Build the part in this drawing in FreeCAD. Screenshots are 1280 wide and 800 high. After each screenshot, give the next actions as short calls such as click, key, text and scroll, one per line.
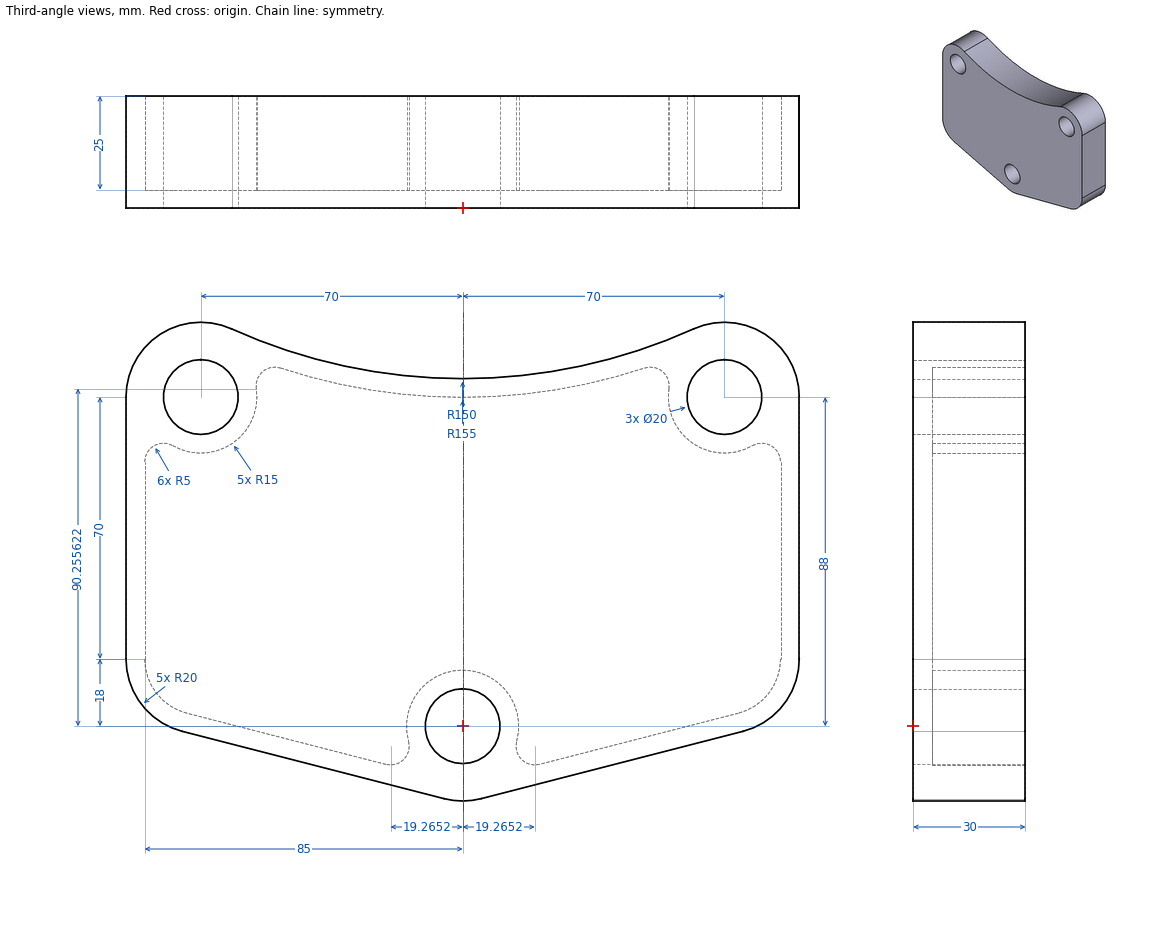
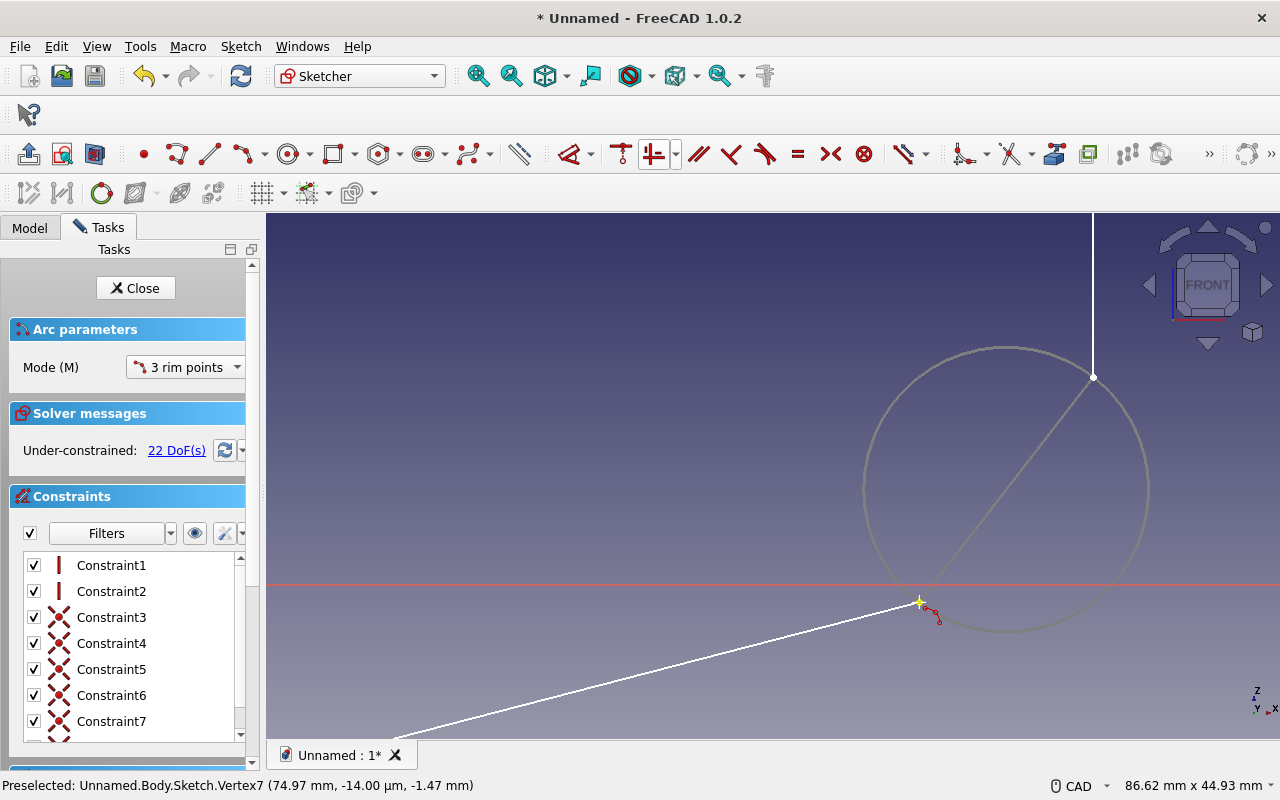
scroll(922, 605, down, 7)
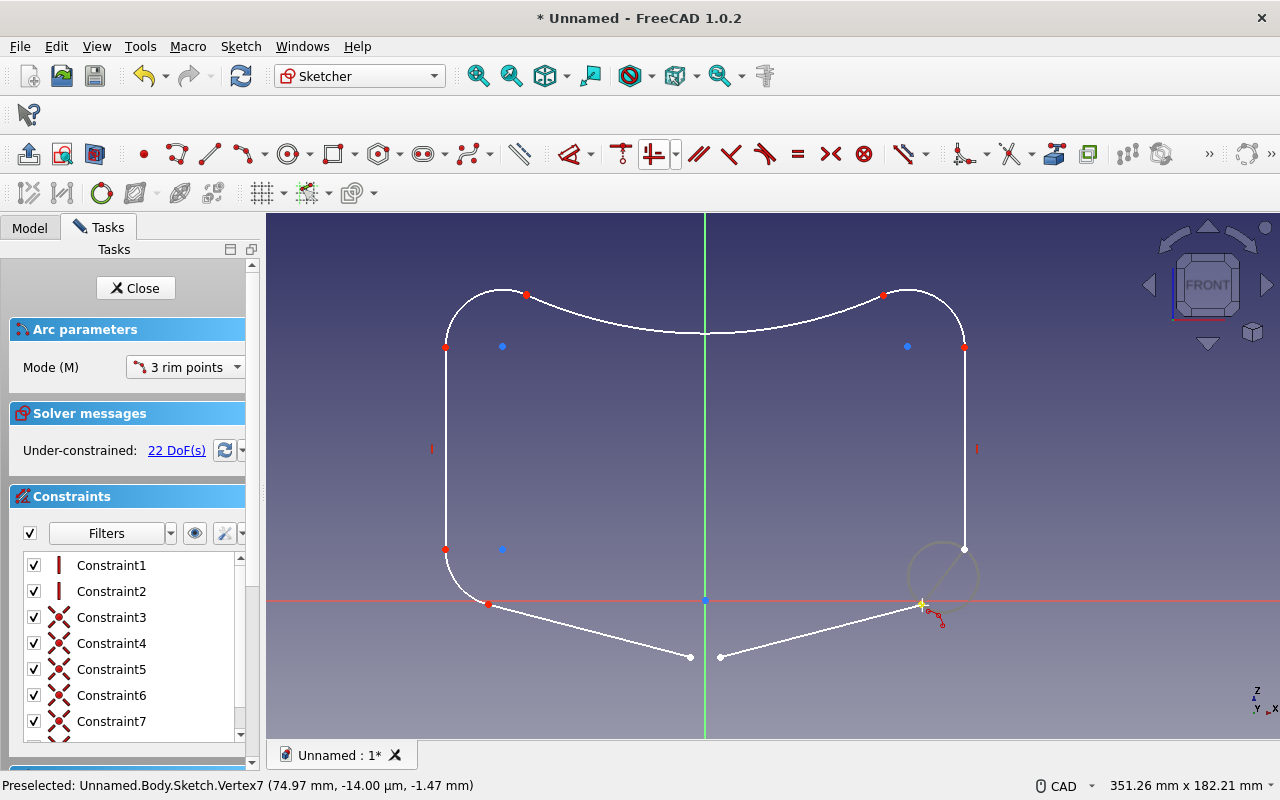
scroll(953, 584, up, 2)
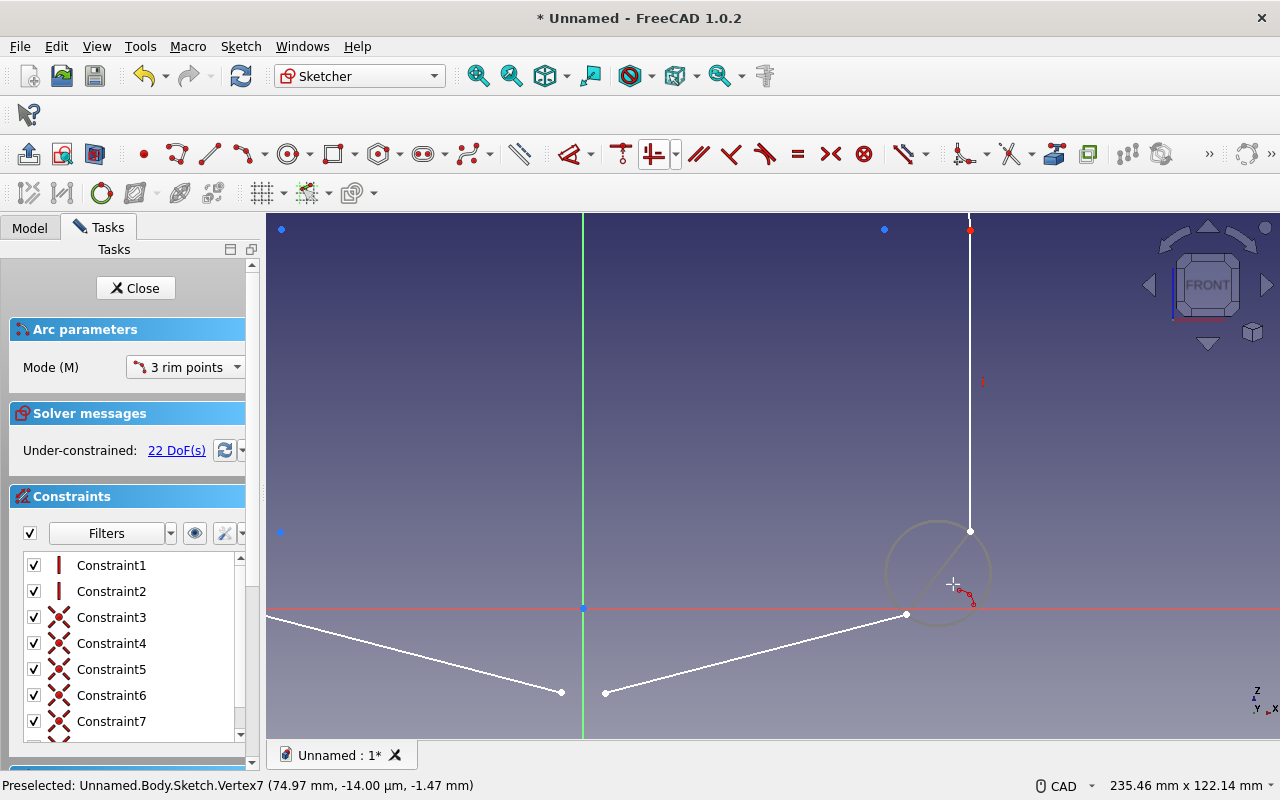
click(953, 584)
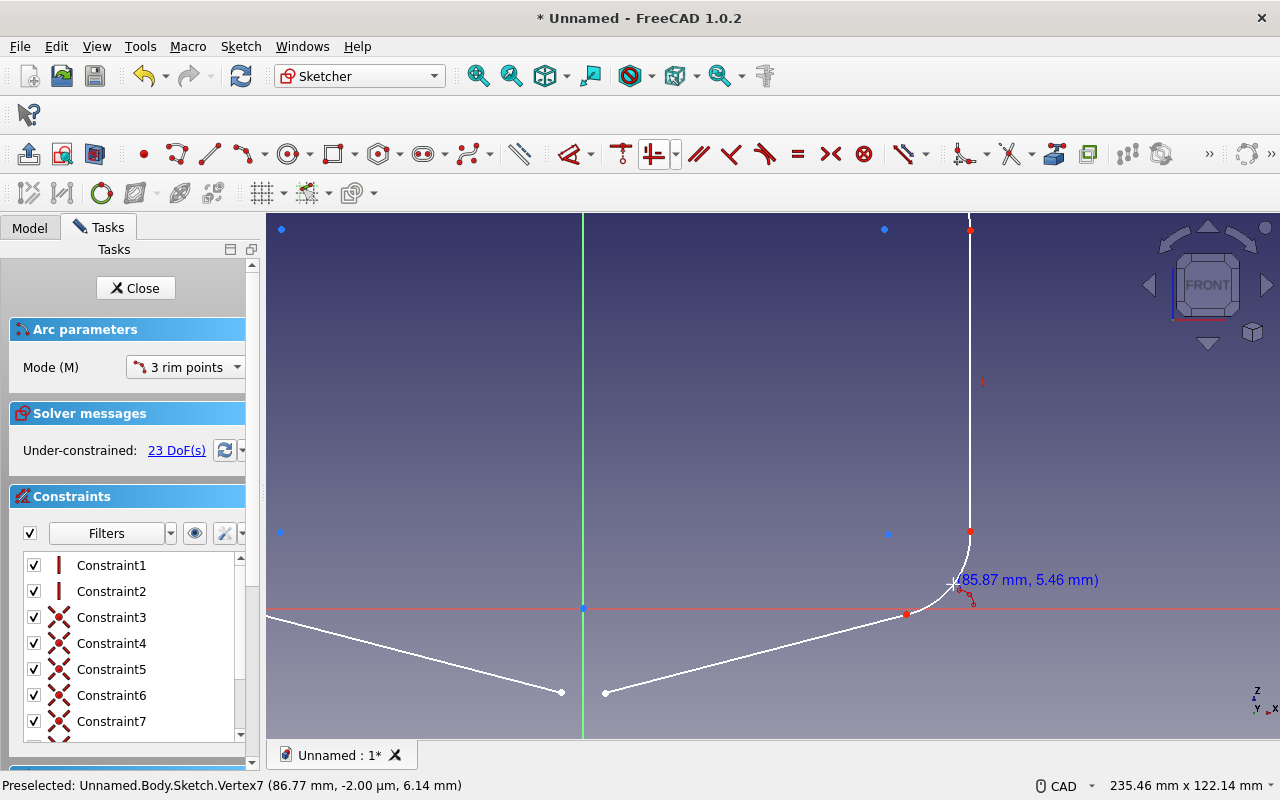
click(605, 693)
click(561, 693)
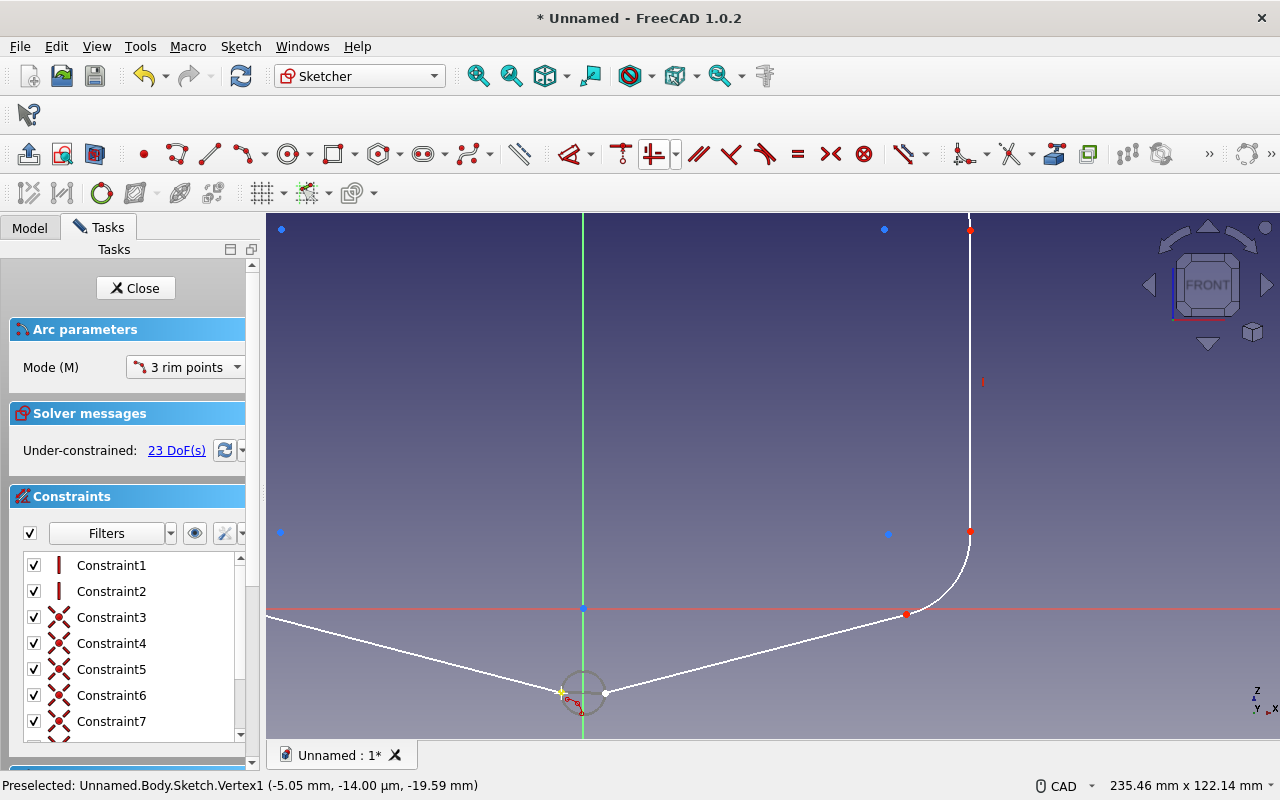
scroll(579, 695, up, 10)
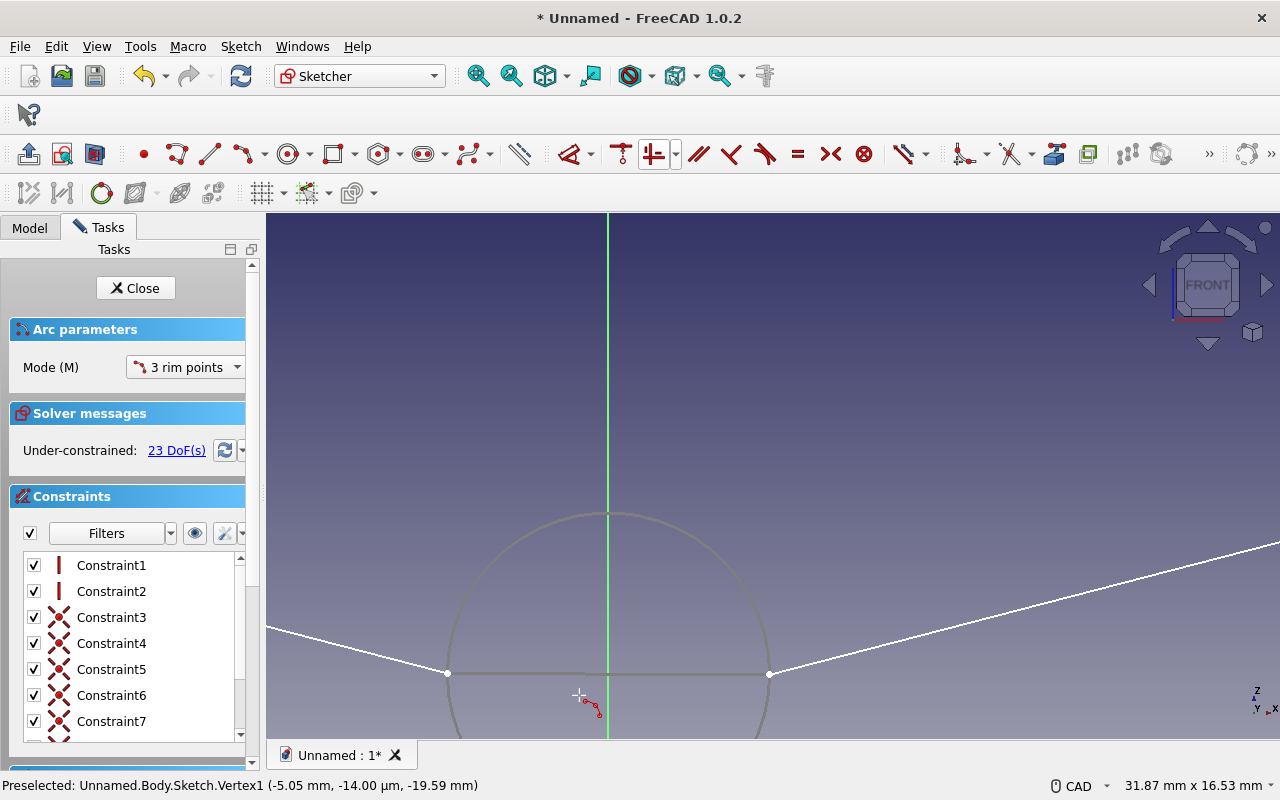
click(576, 686)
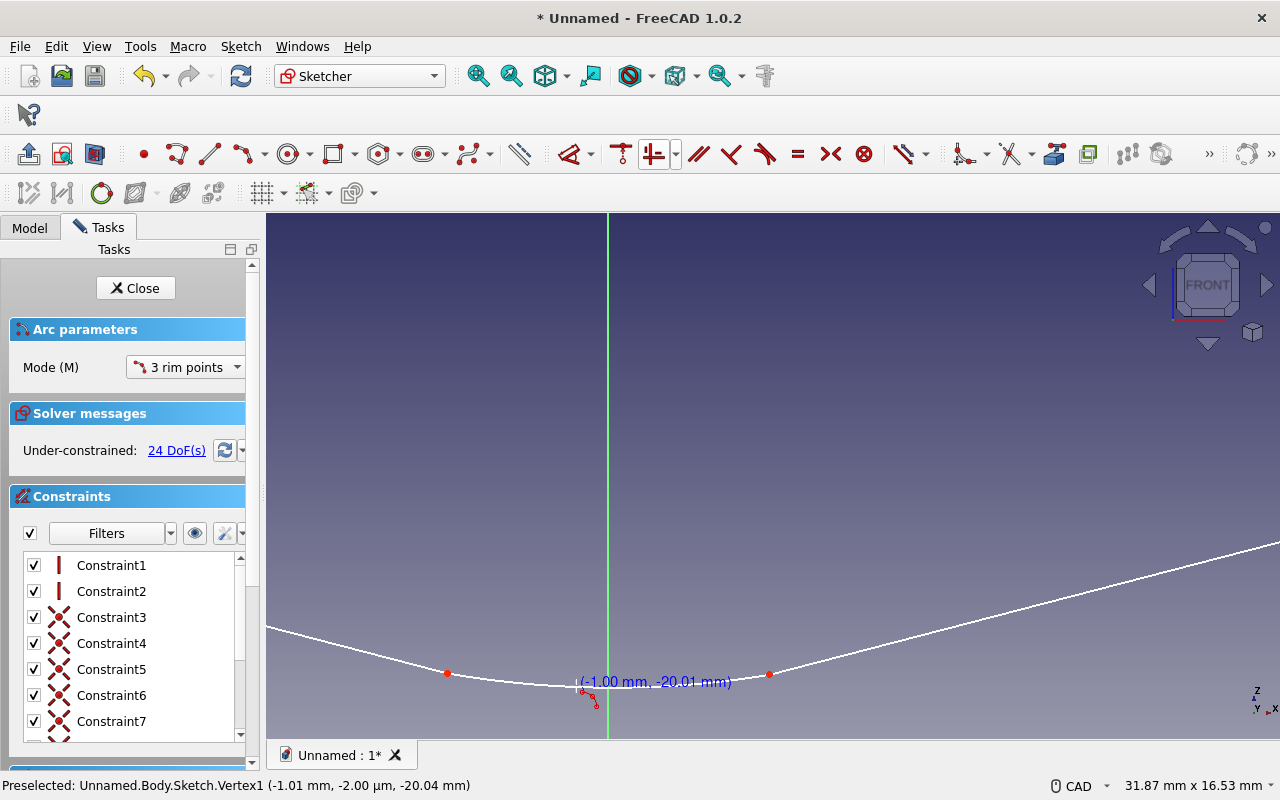
click(288, 154)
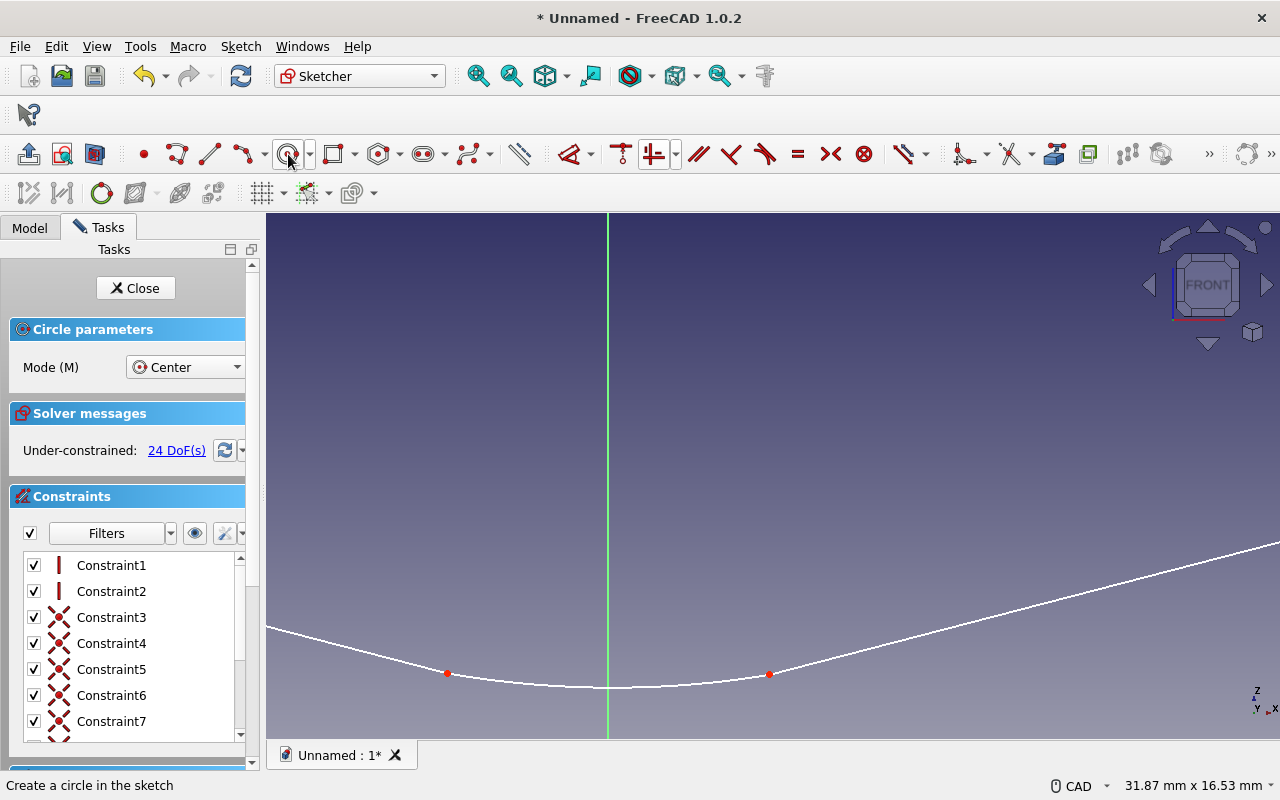
scroll(714, 655, down, 12)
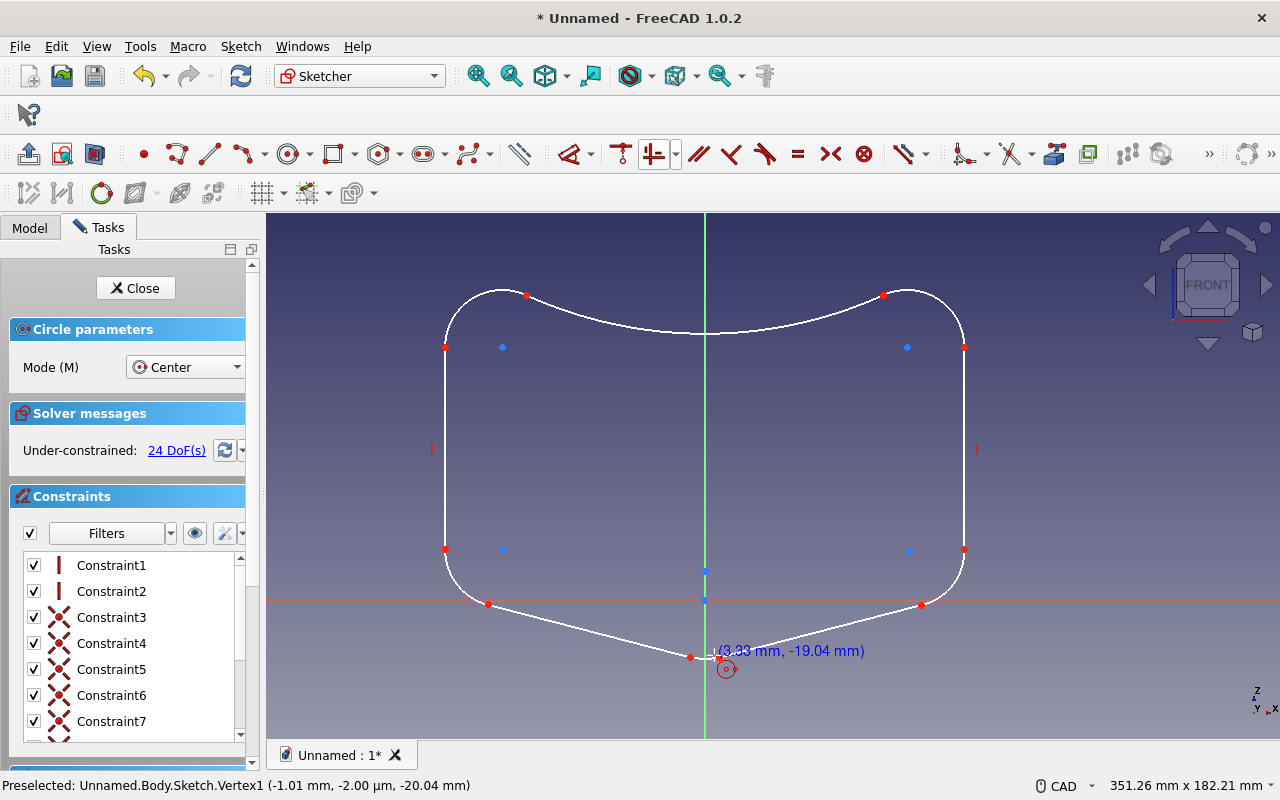
click(907, 347)
move(927, 326)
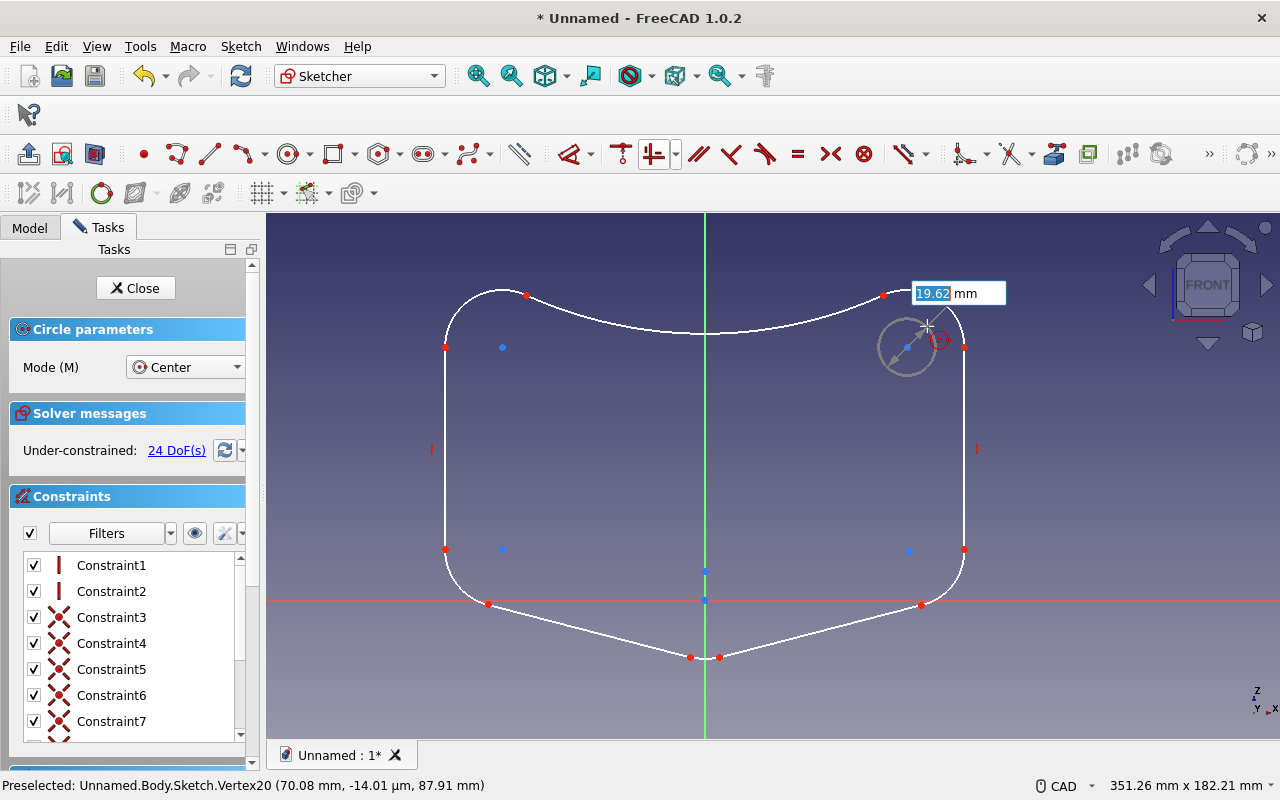
text(20)
key(Return)